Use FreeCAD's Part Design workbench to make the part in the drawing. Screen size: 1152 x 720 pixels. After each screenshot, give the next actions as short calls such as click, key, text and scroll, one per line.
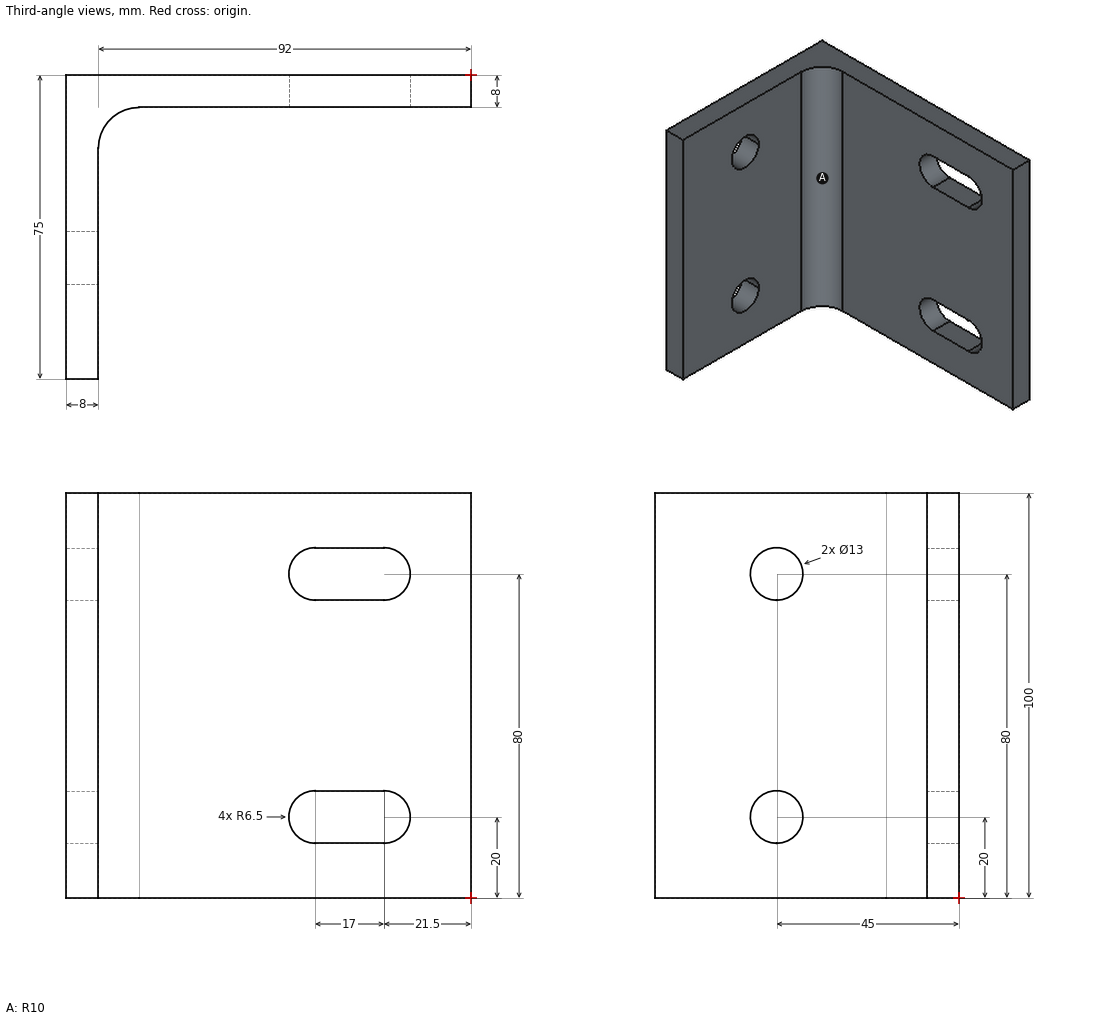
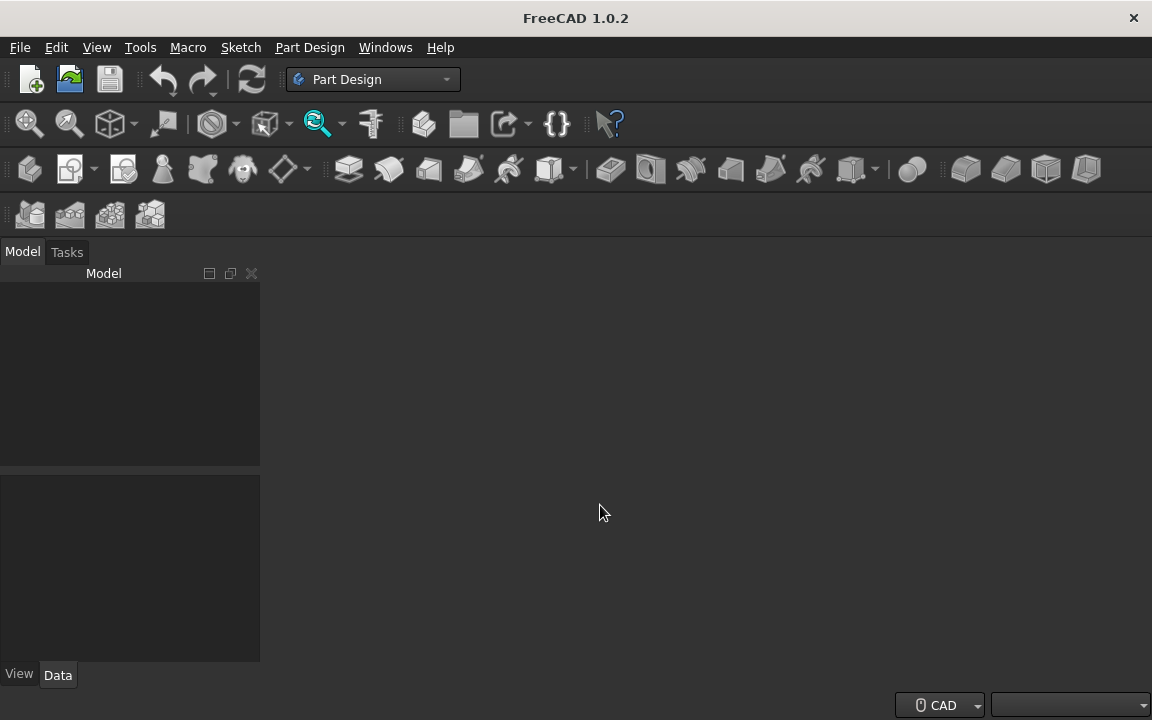
key(ctrl+n)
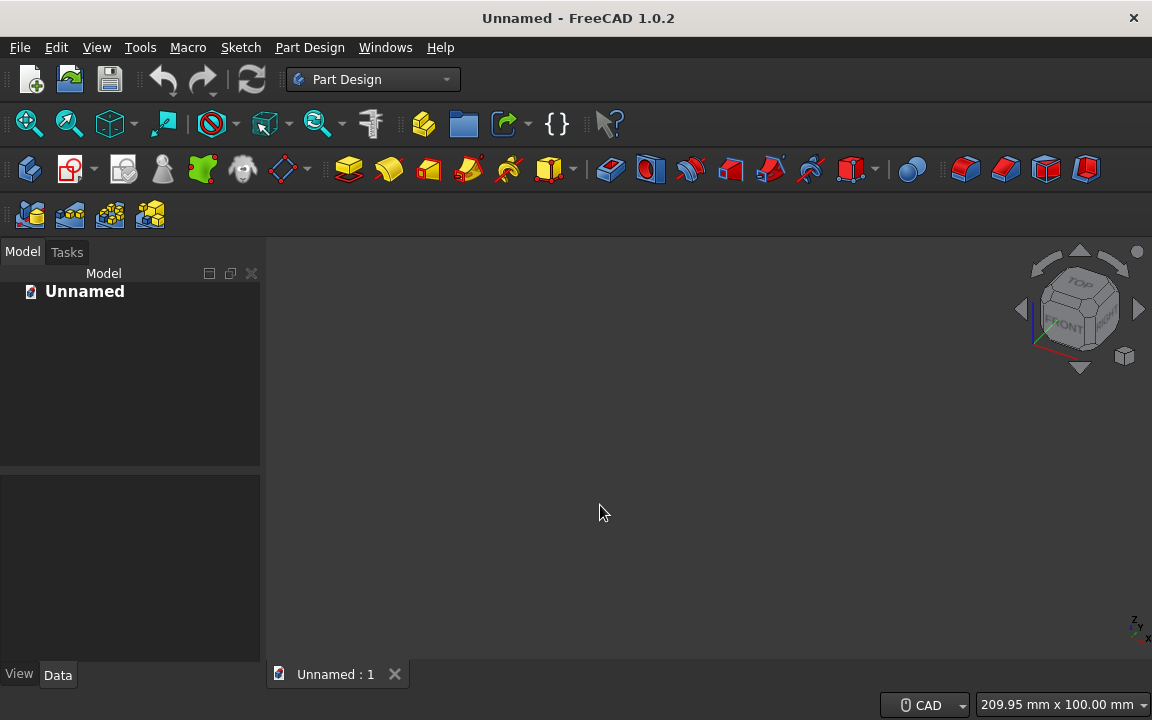
click(70, 170)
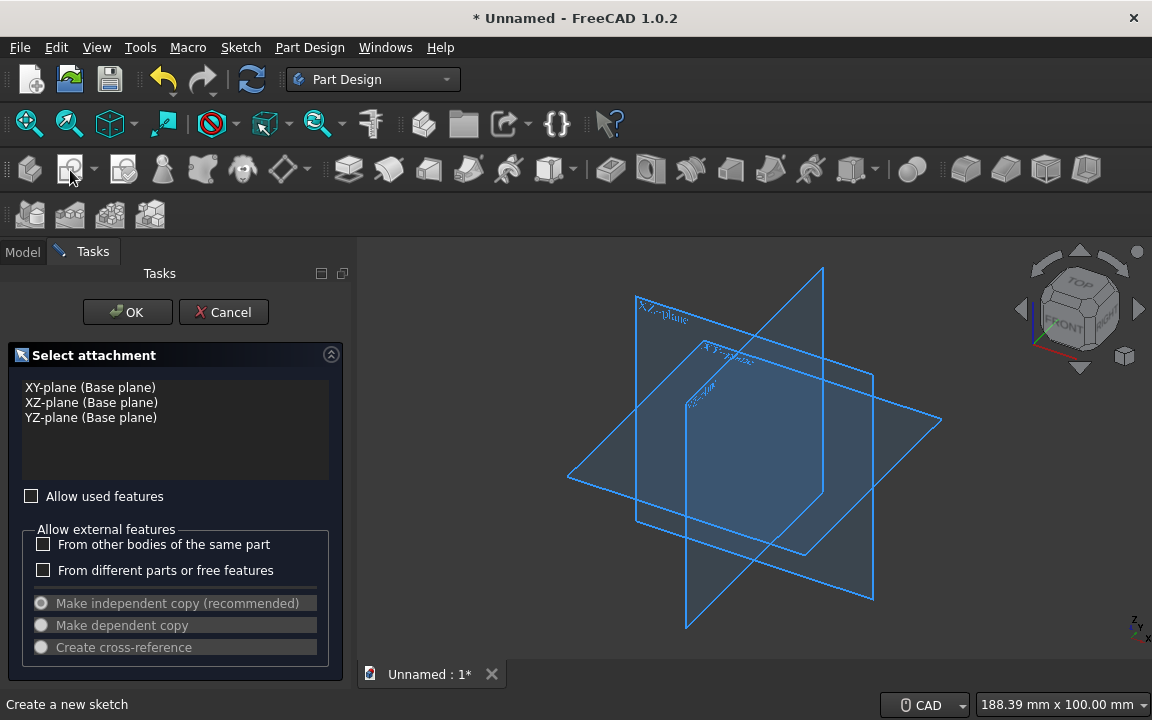
click(82, 388)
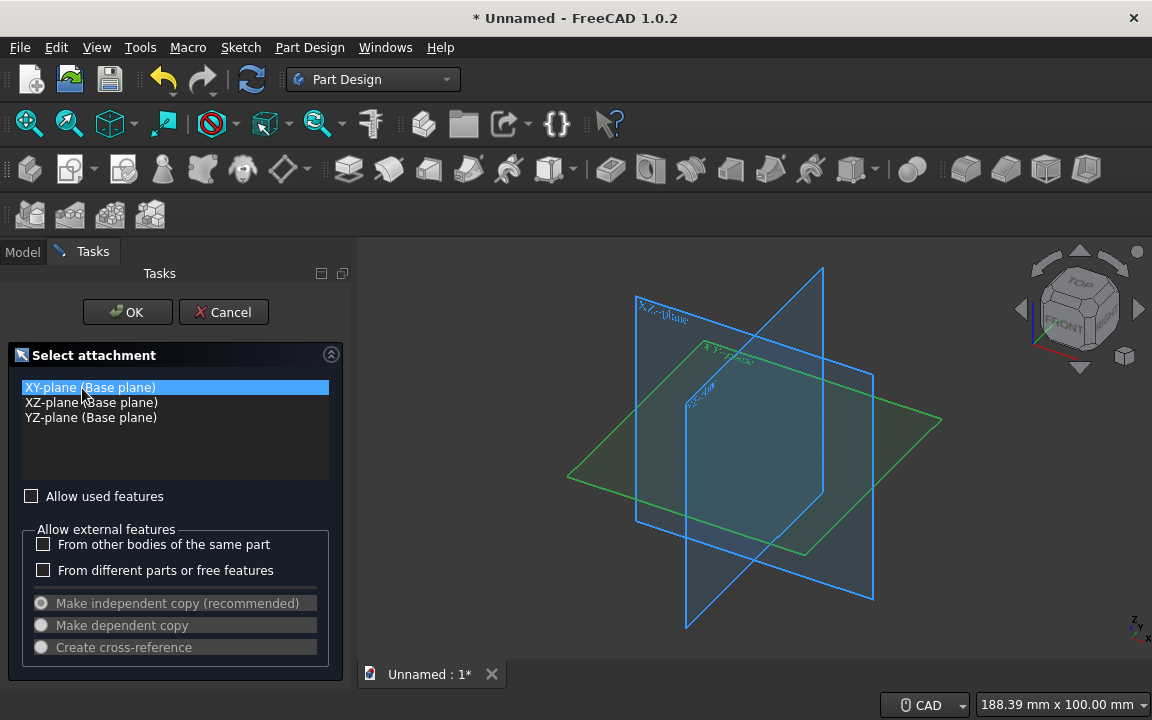
click(128, 312)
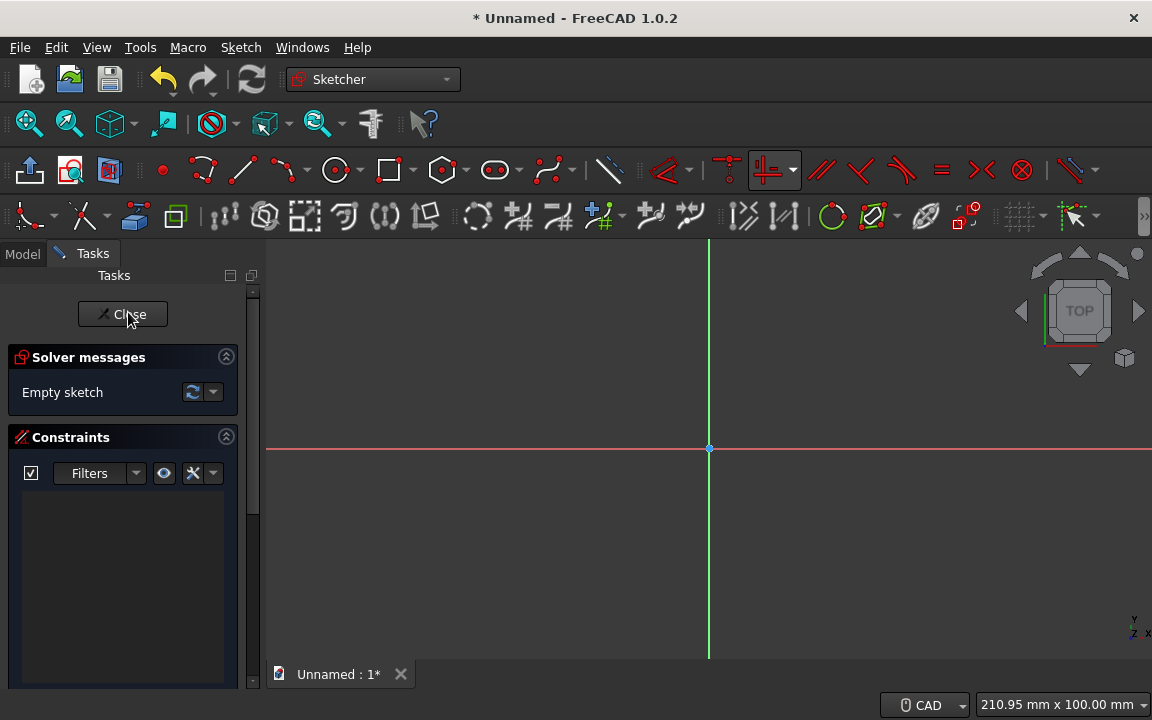
scroll(928, 267, down, 2)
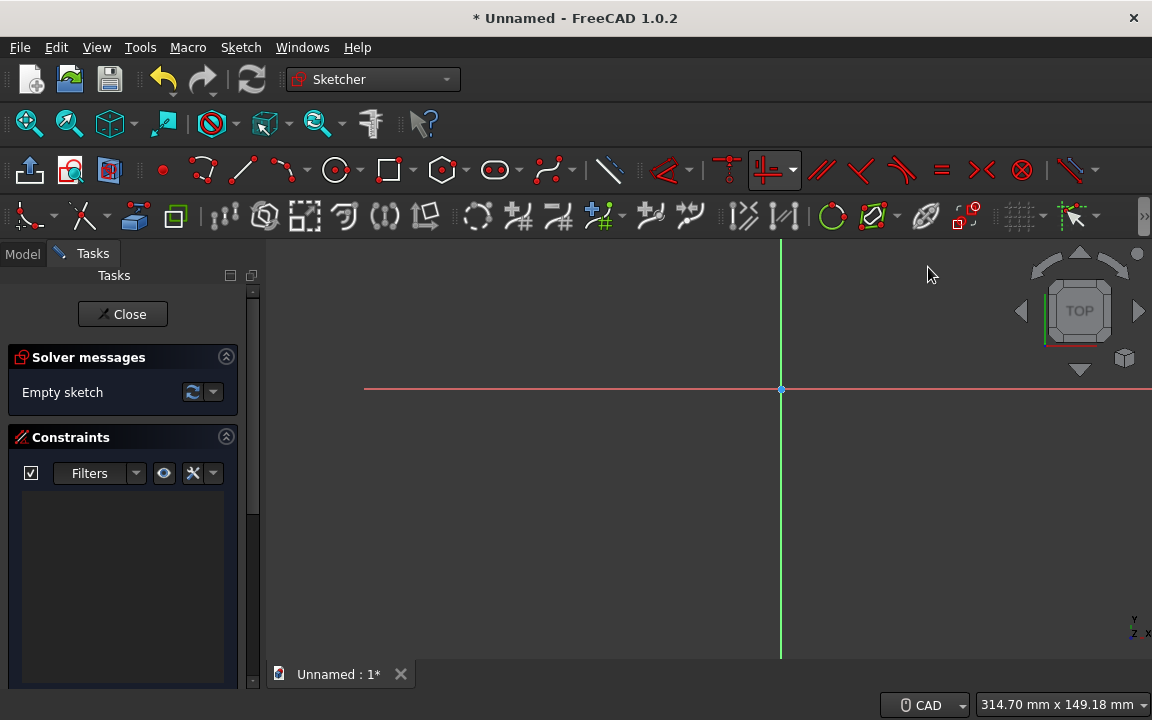
key(g)
key(m)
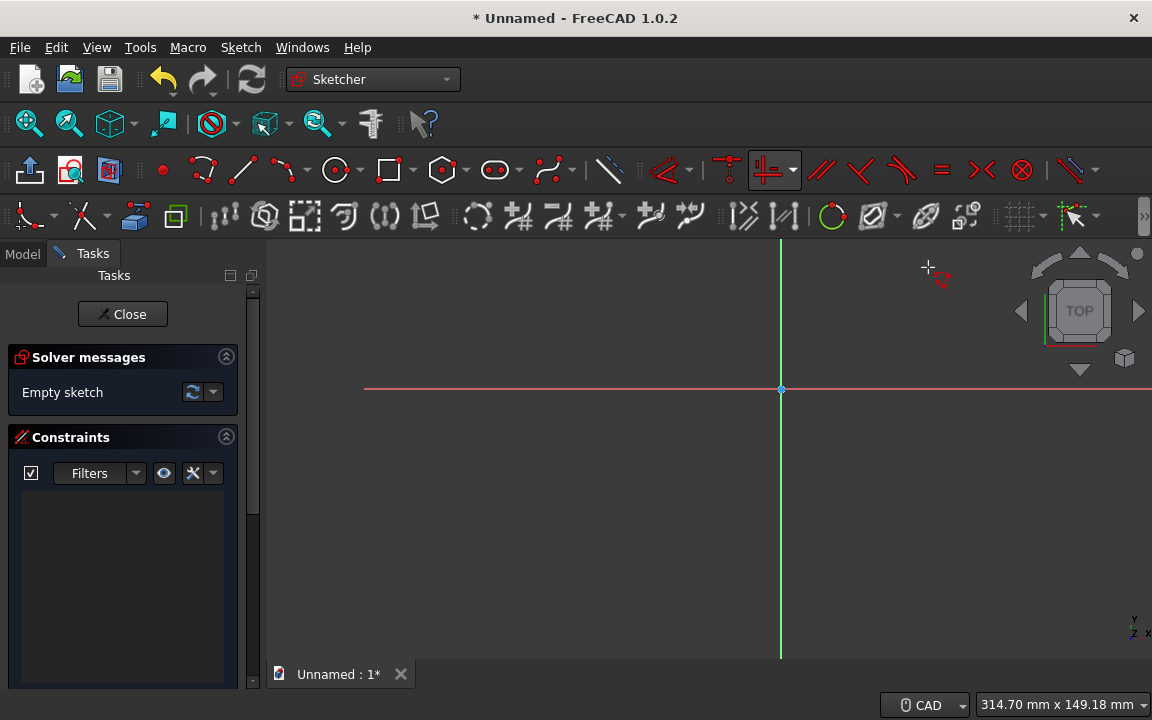
click(781, 389)
click(500, 398)
click(500, 600)
click(522, 600)
click(522, 412)
click(772, 412)
click(781, 389)
key(Escape)
key(Escape)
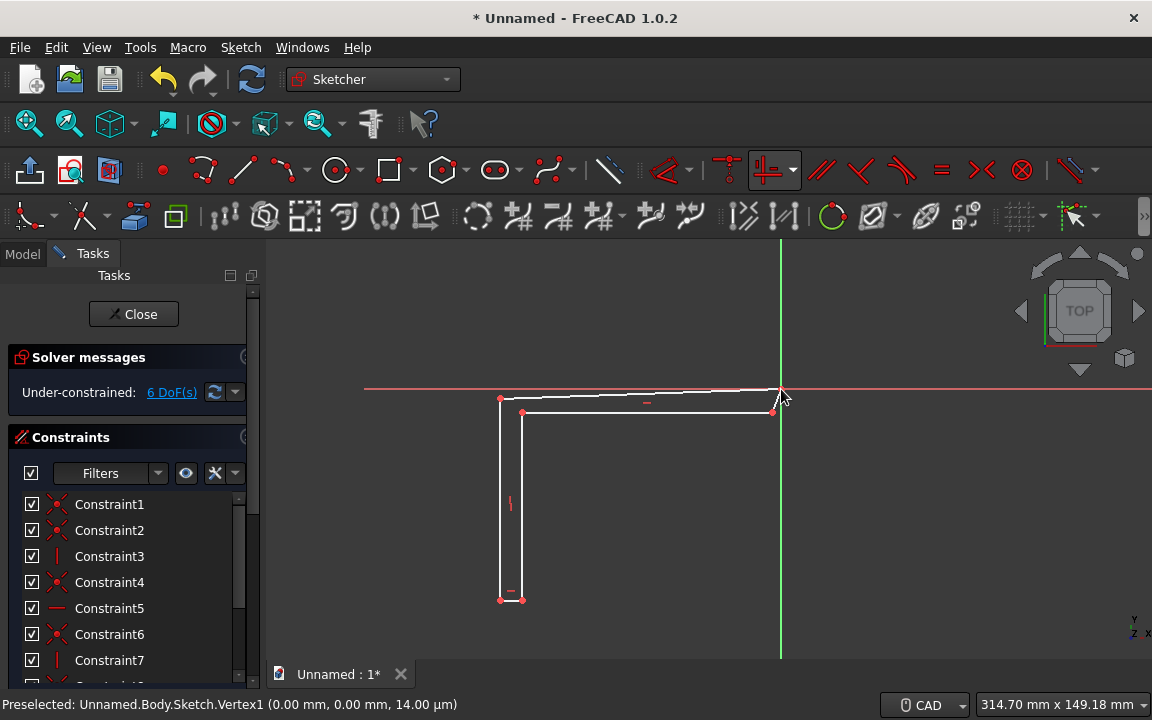
click(697, 392)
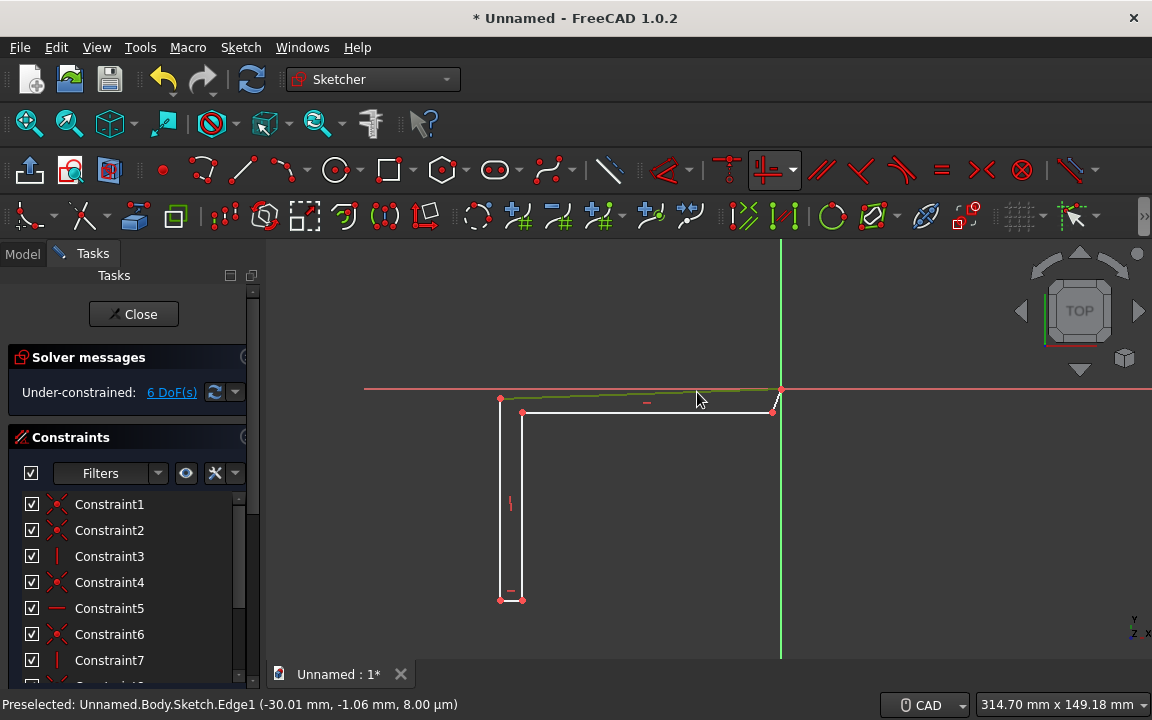
key(h)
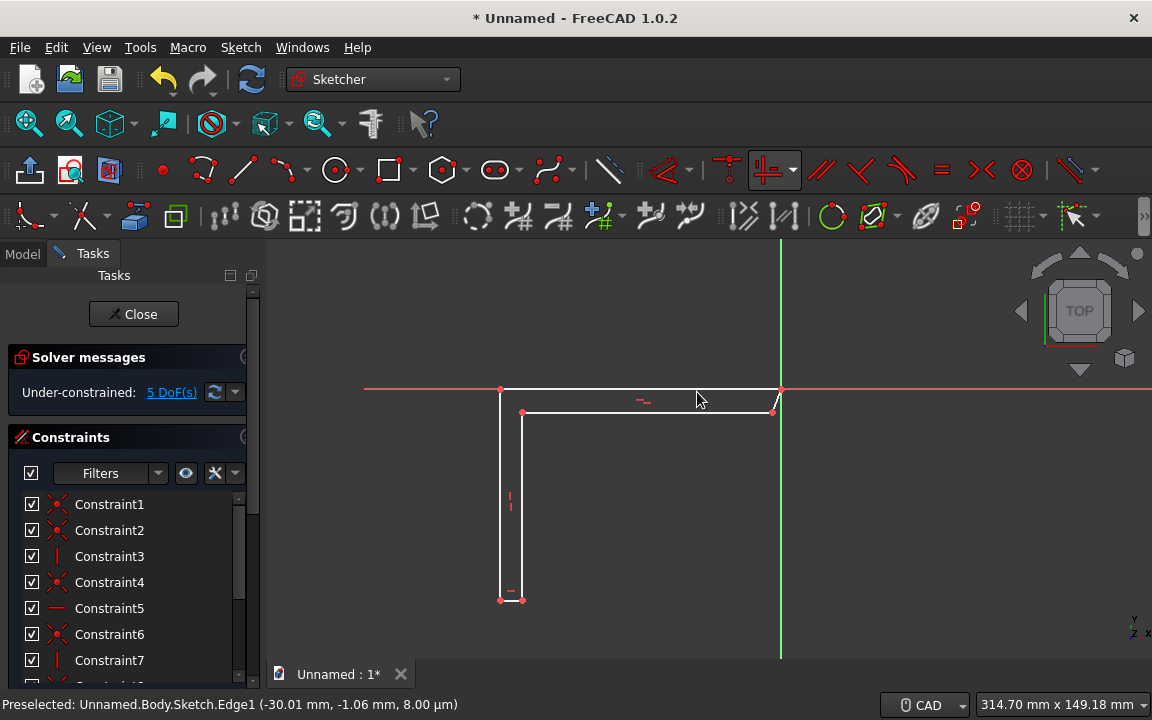
scroll(778, 399, up, 2)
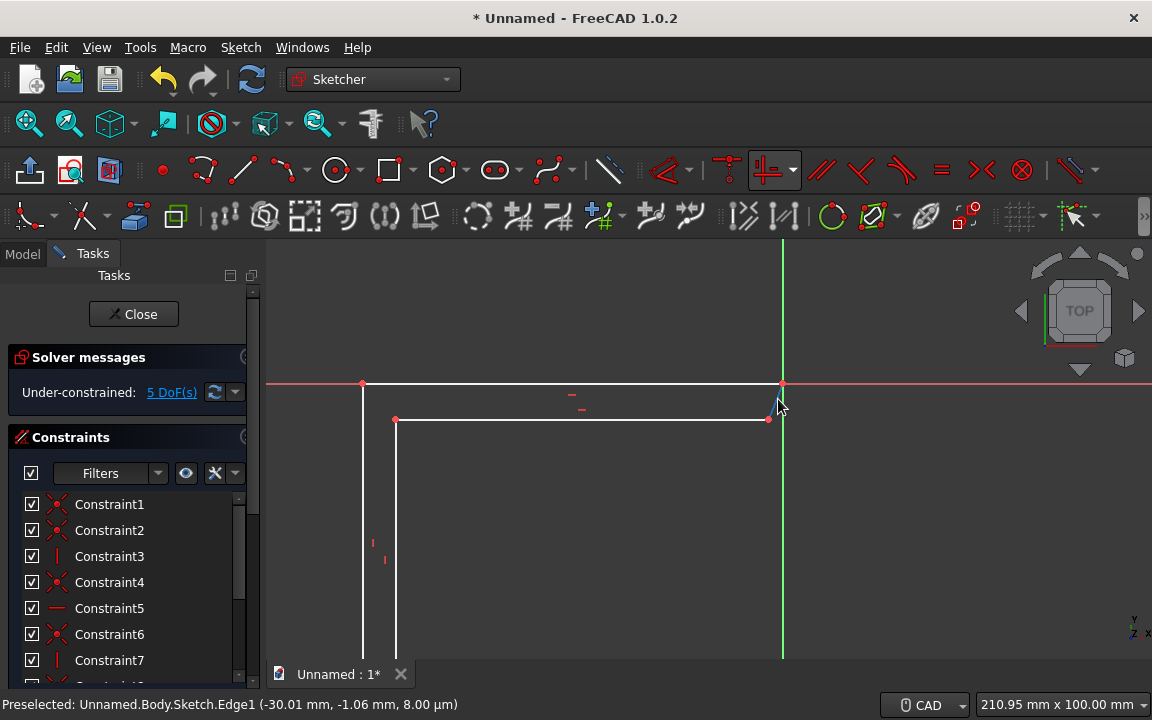
click(777, 398)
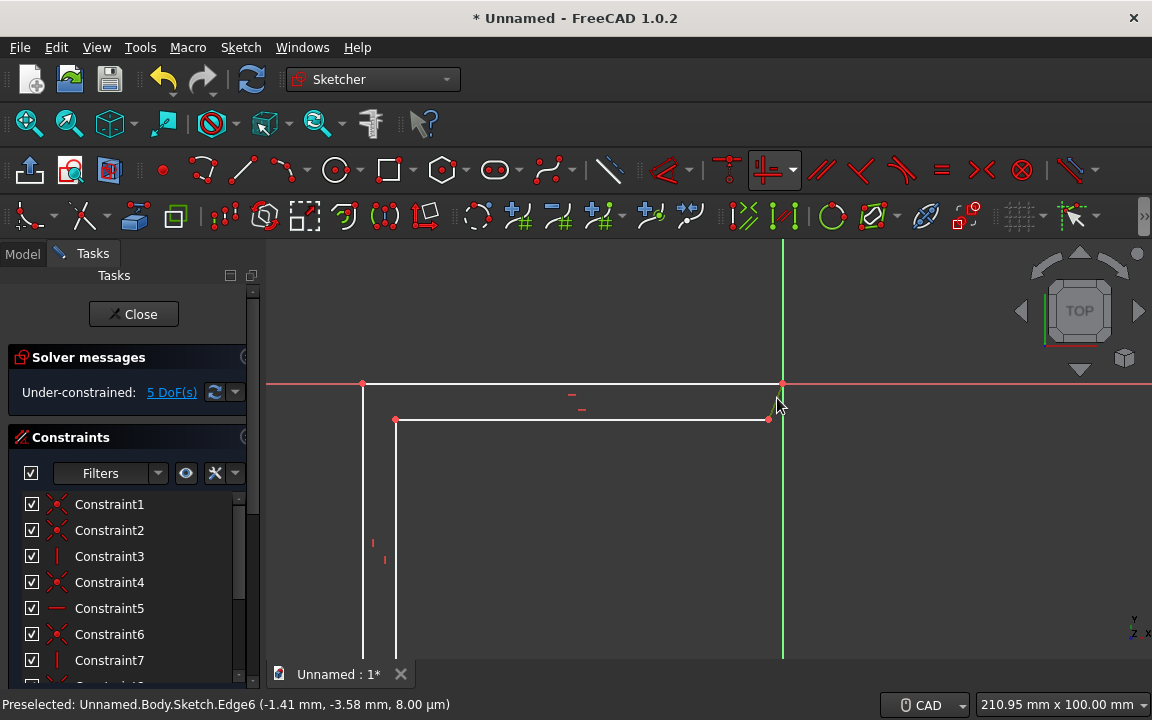
key(v)